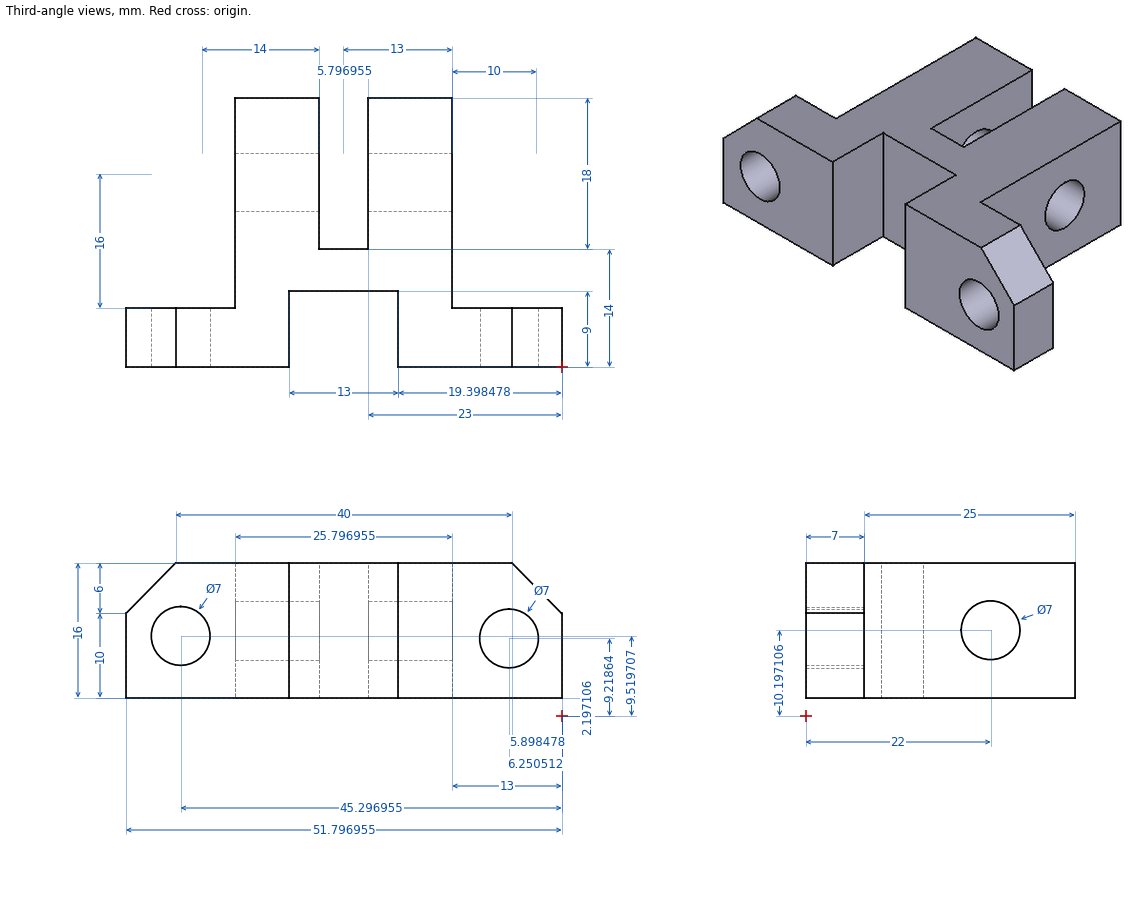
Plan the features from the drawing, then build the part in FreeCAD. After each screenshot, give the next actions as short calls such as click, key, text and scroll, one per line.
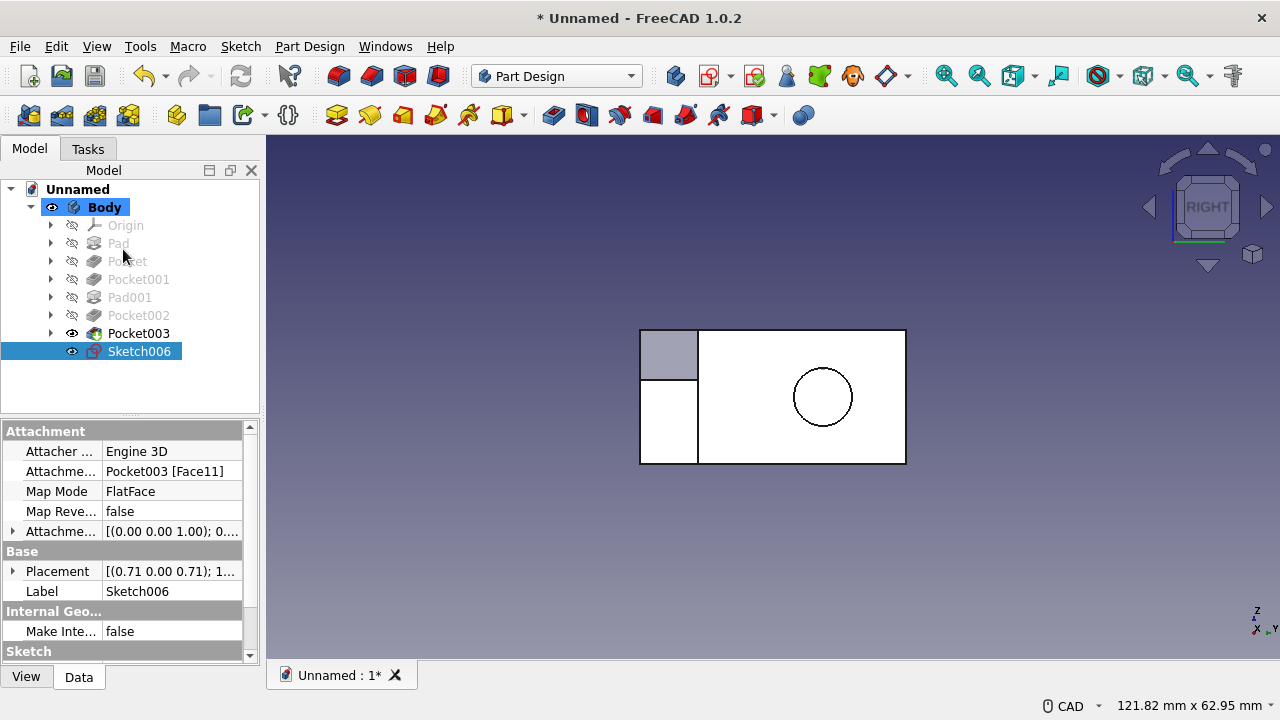
click(554, 116)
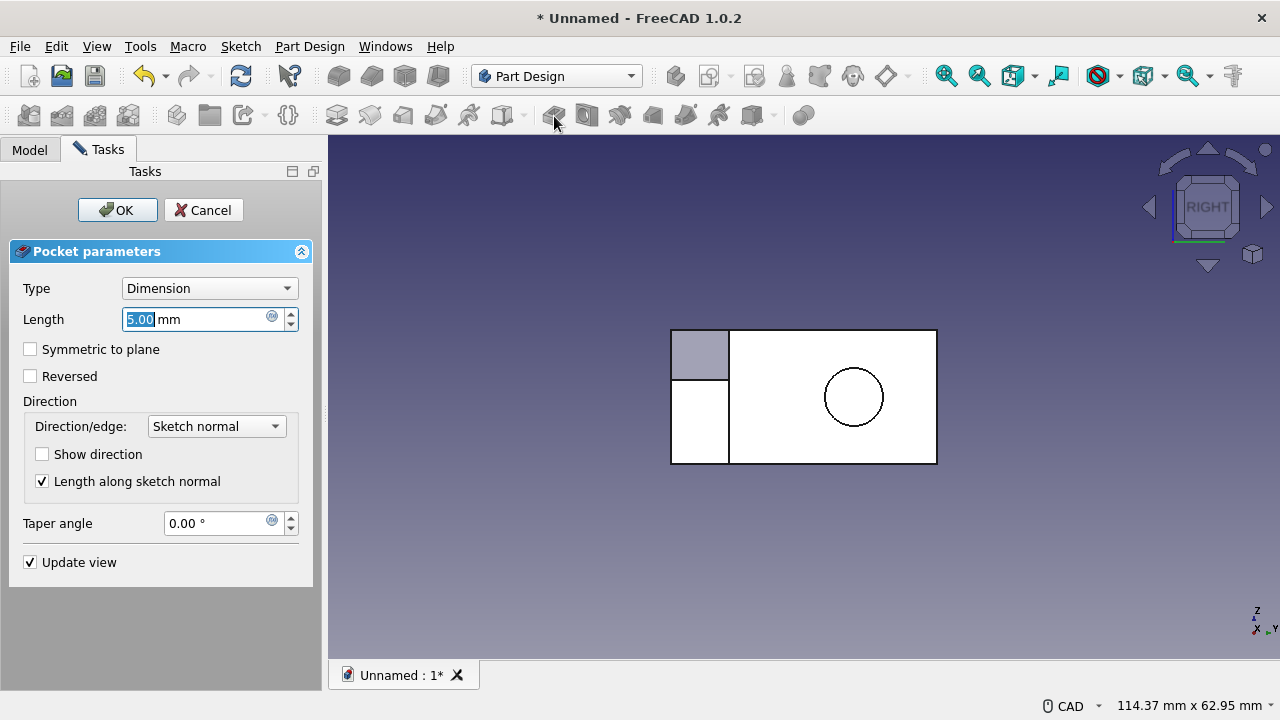
text(14)
key(Tab)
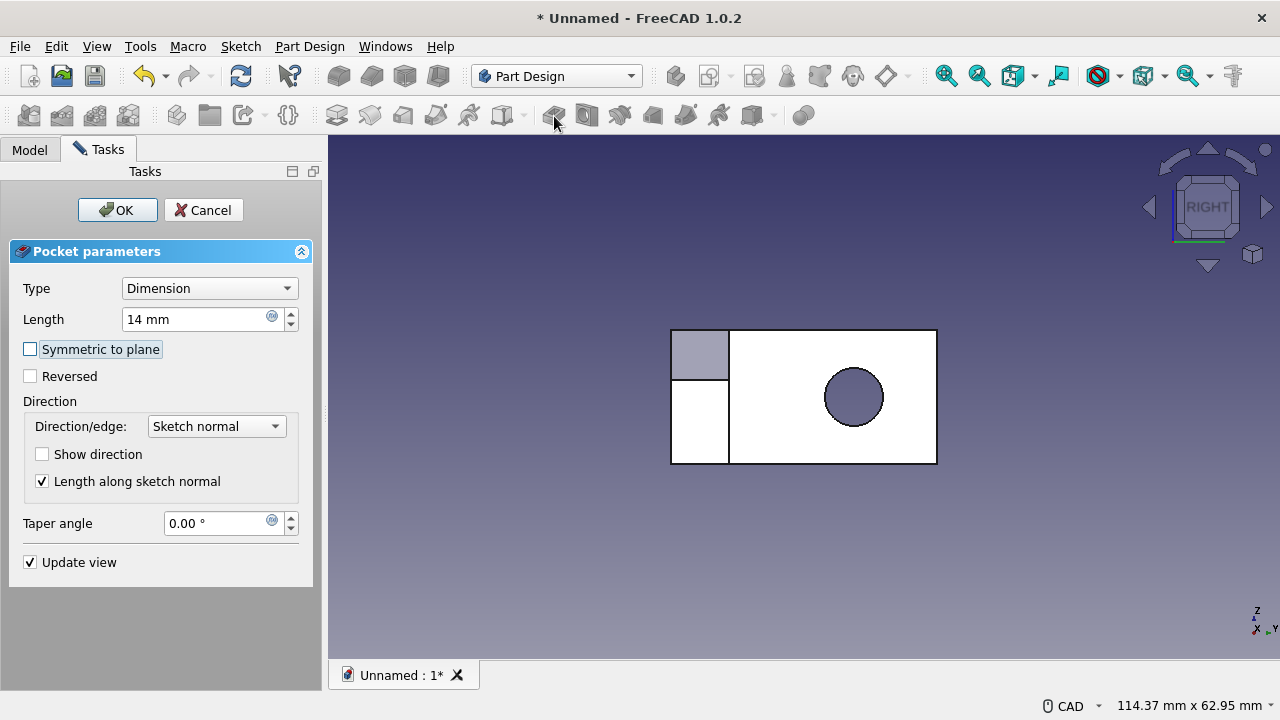
click(118, 210)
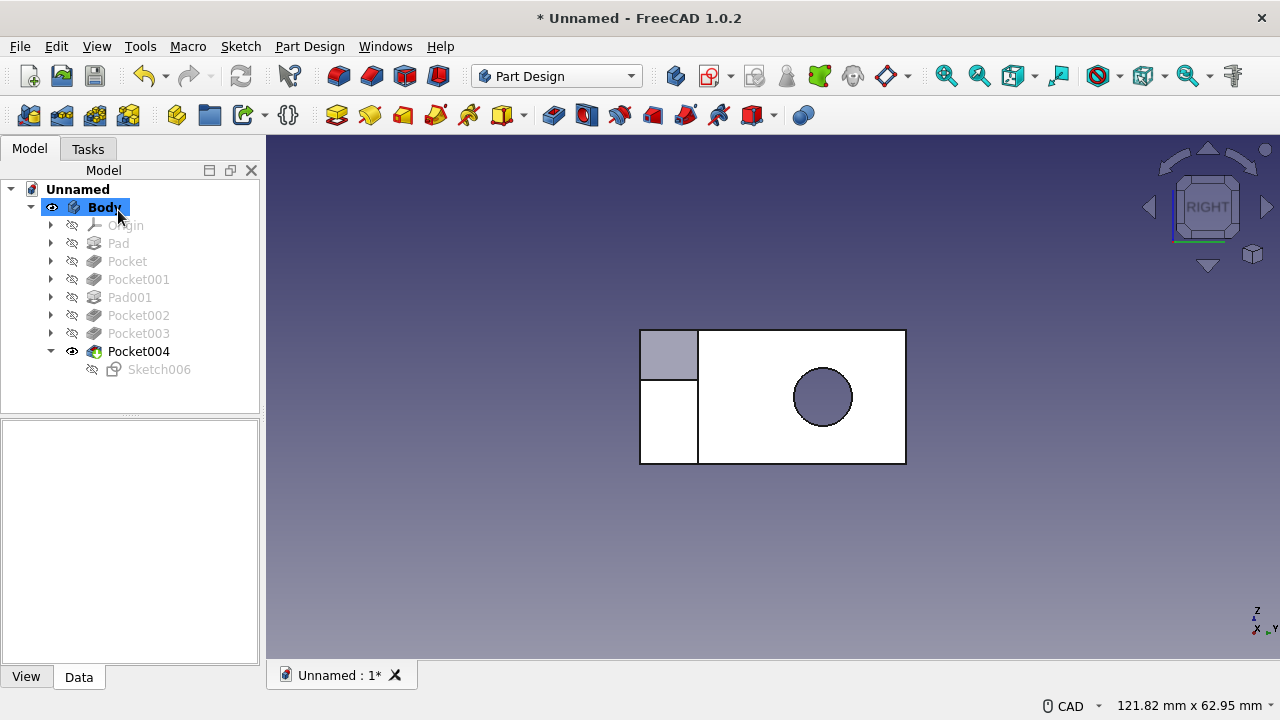
click(947, 76)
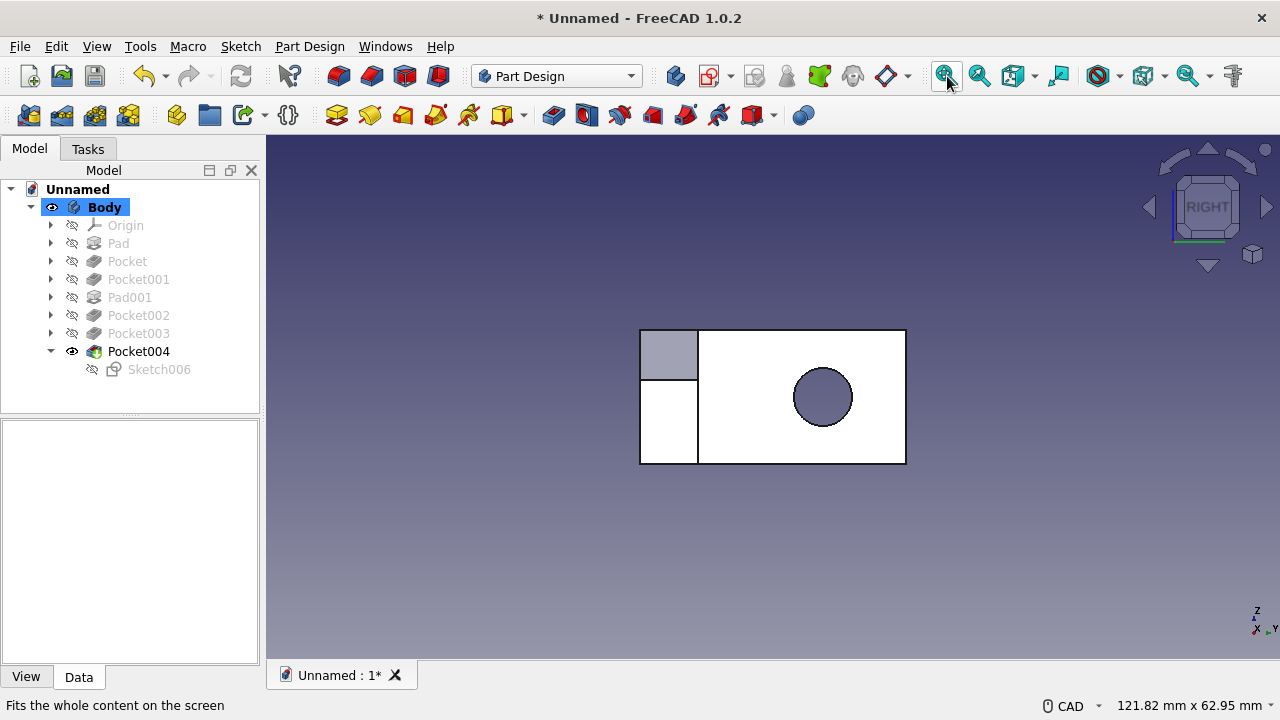
key(0)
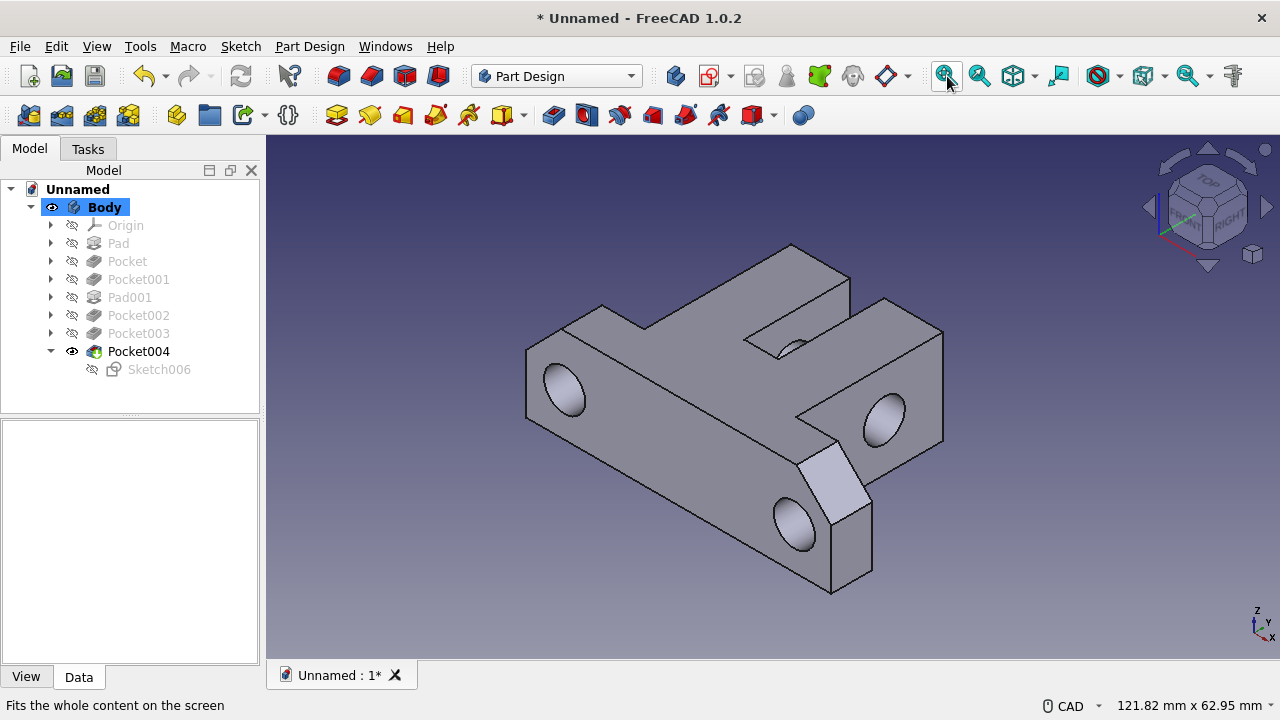
click(753, 392)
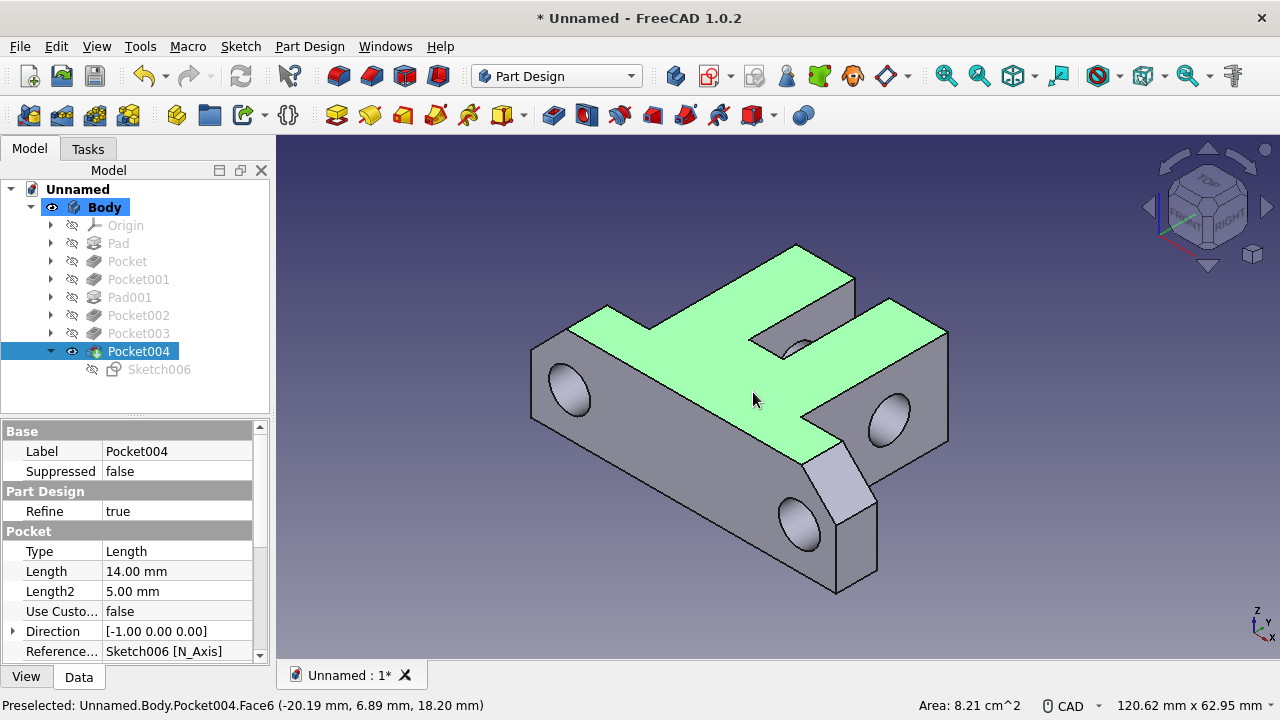
click(708, 76)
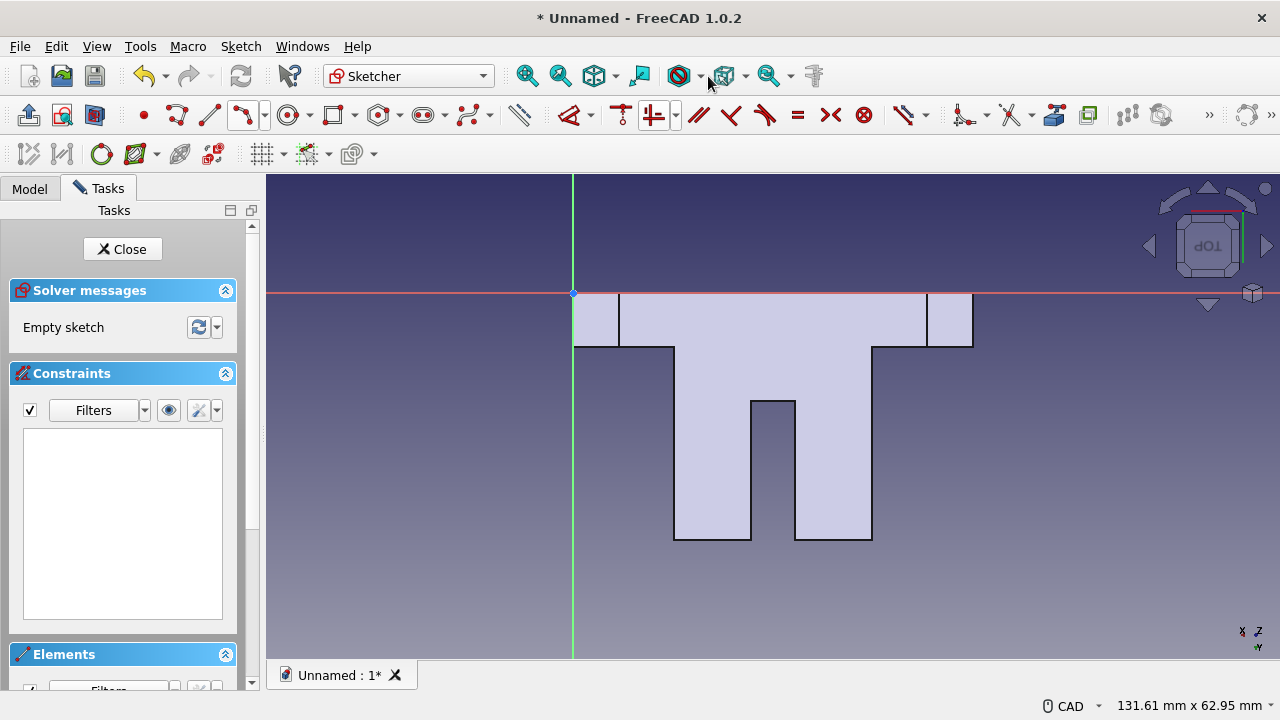
scroll(693, 256, up, 4)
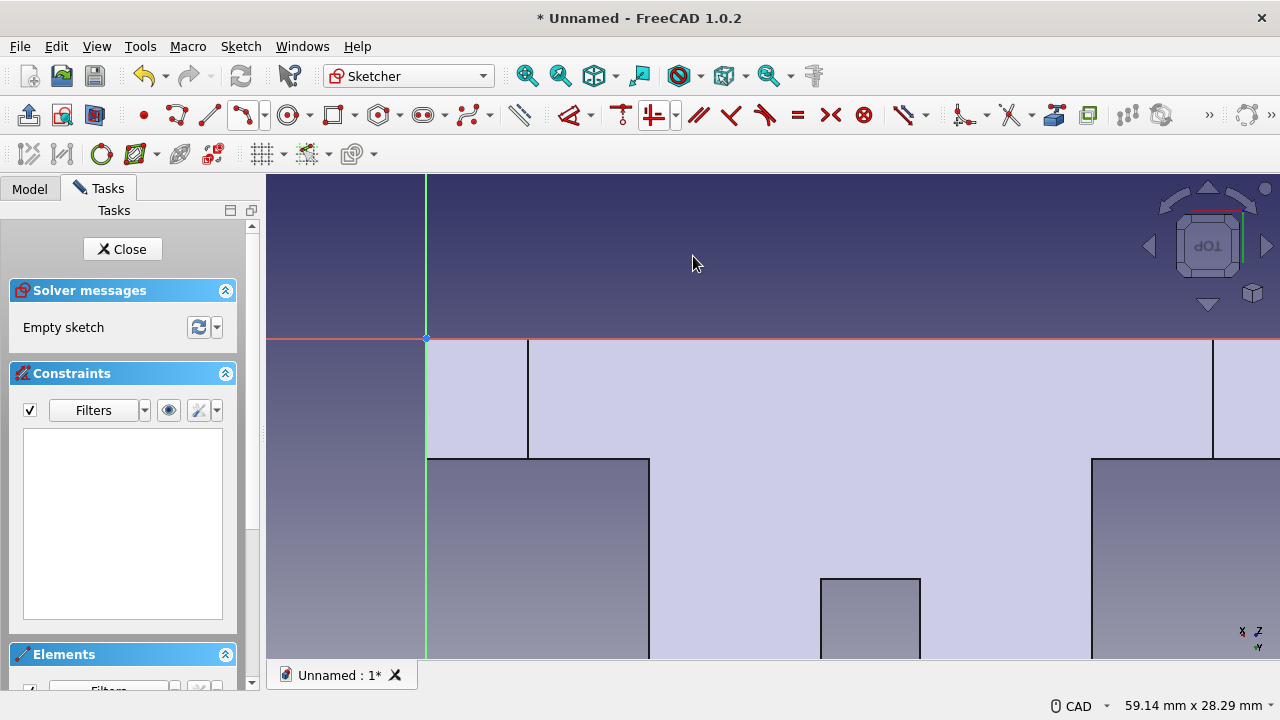
click(332, 116)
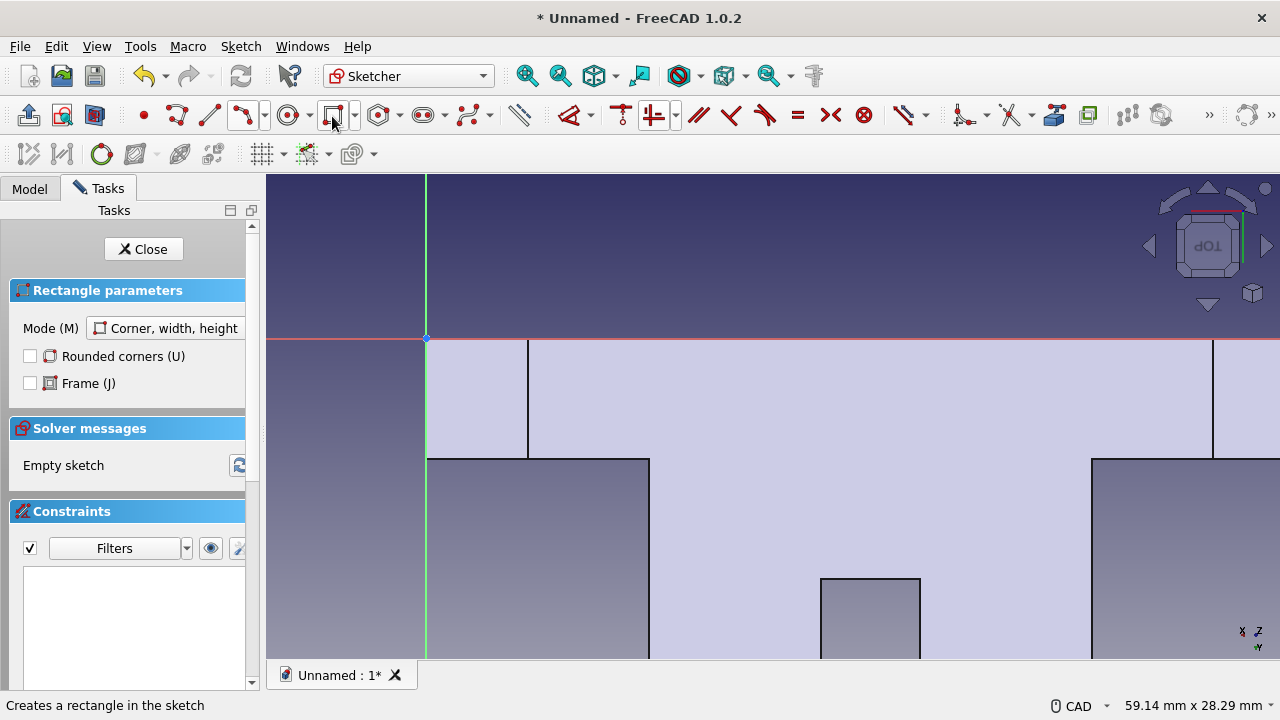
click(759, 339)
click(982, 493)
key(Escape)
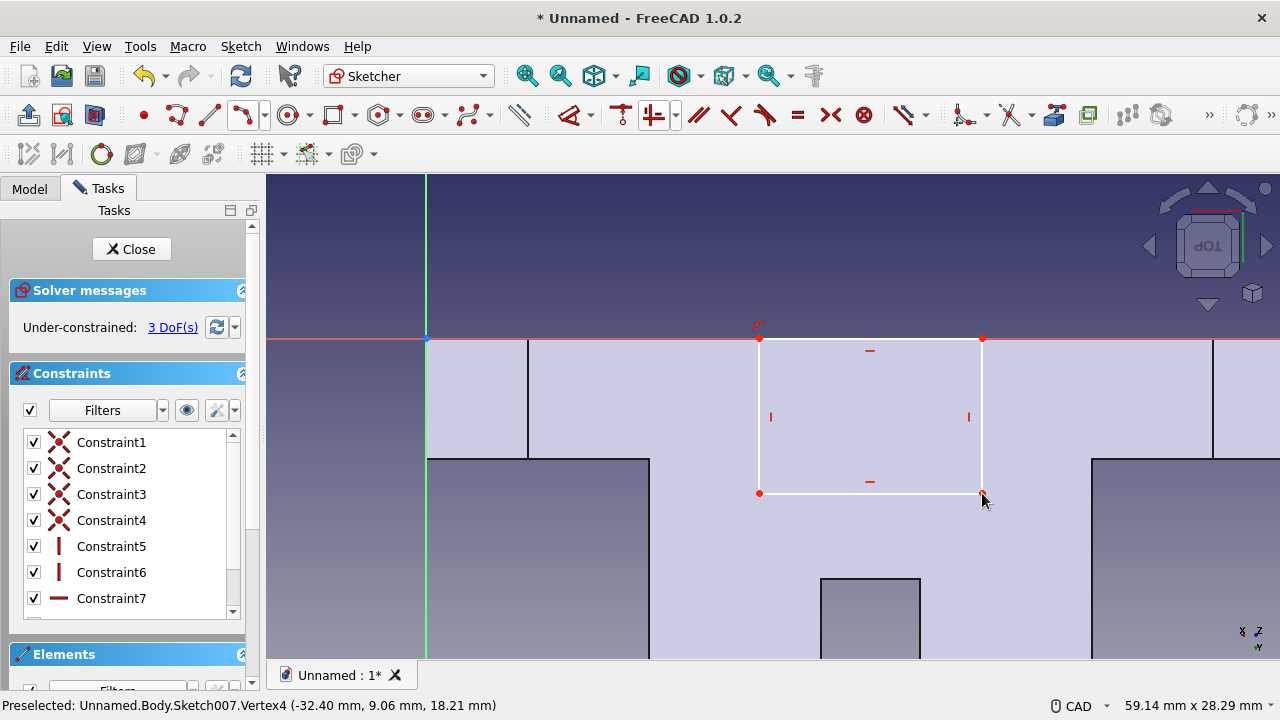
click(568, 116)